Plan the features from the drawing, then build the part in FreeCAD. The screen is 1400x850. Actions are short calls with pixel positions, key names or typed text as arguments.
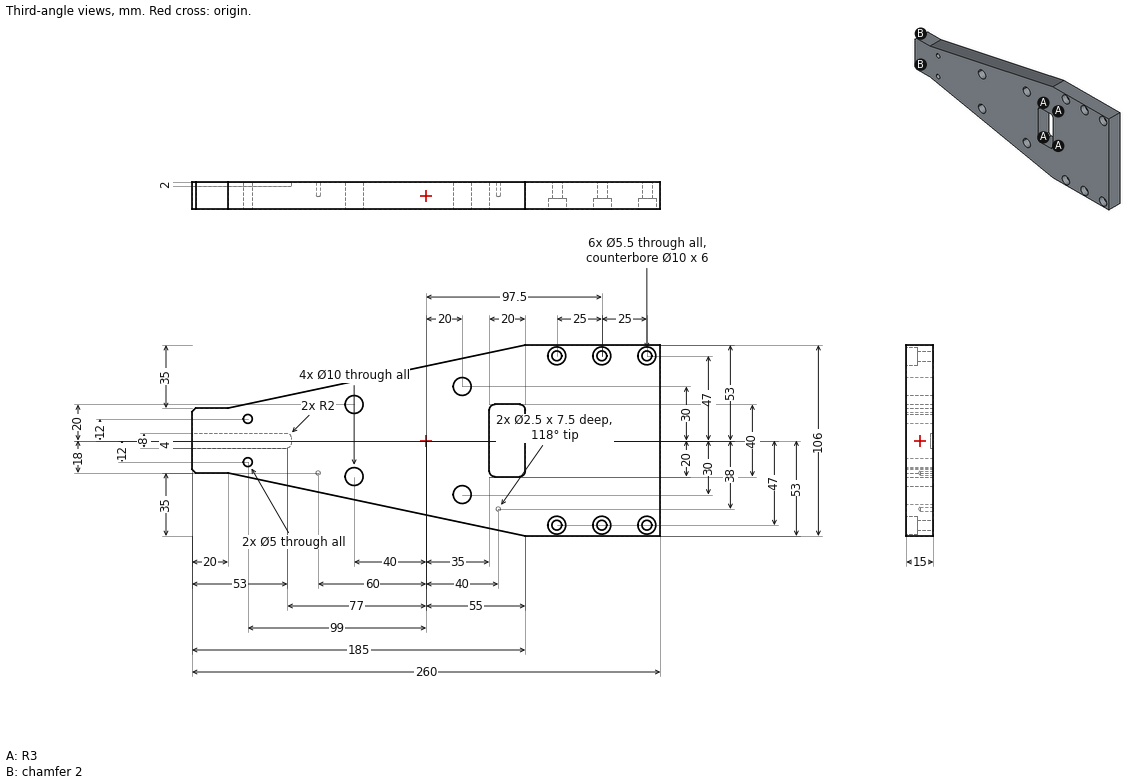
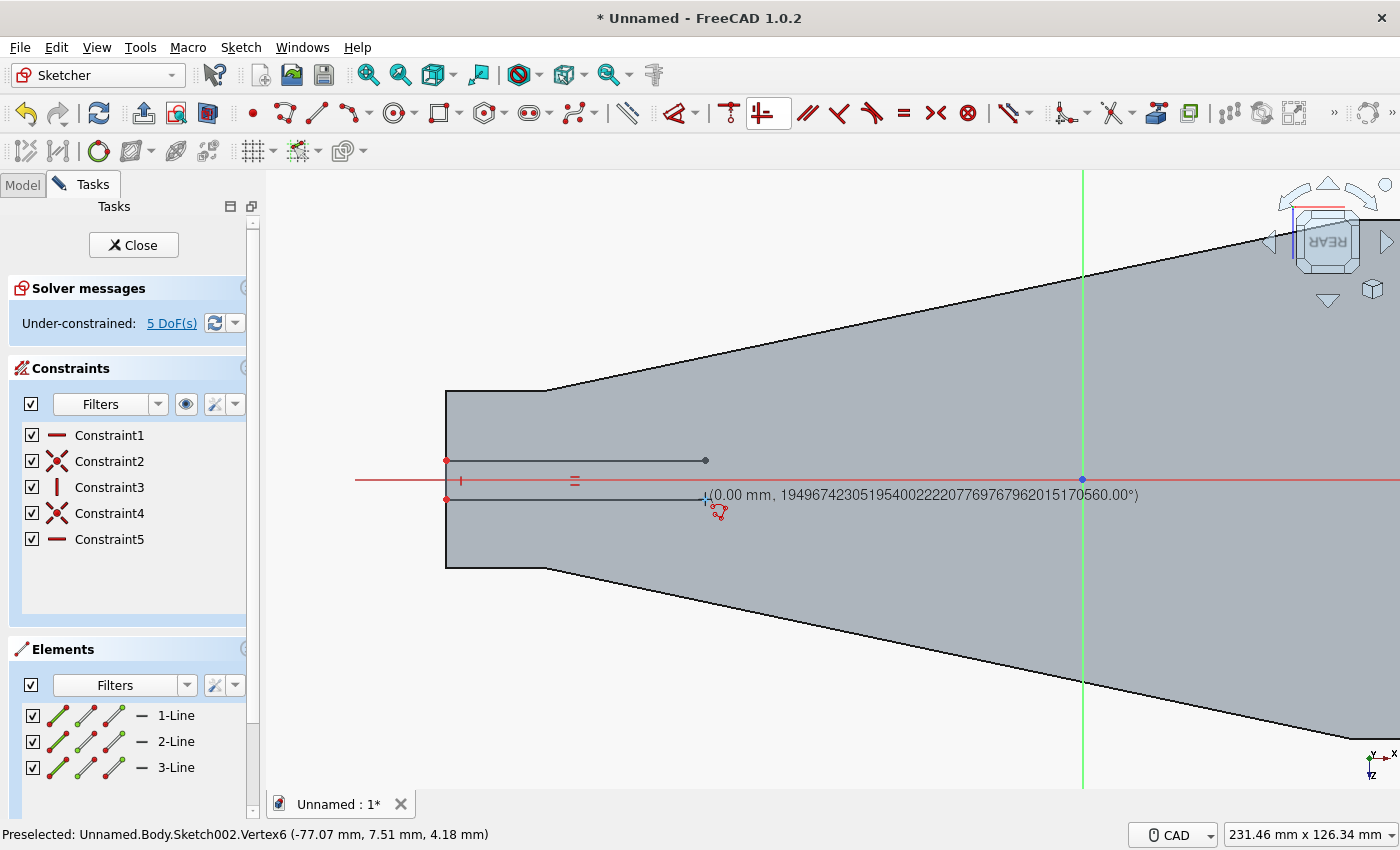
click(318, 114)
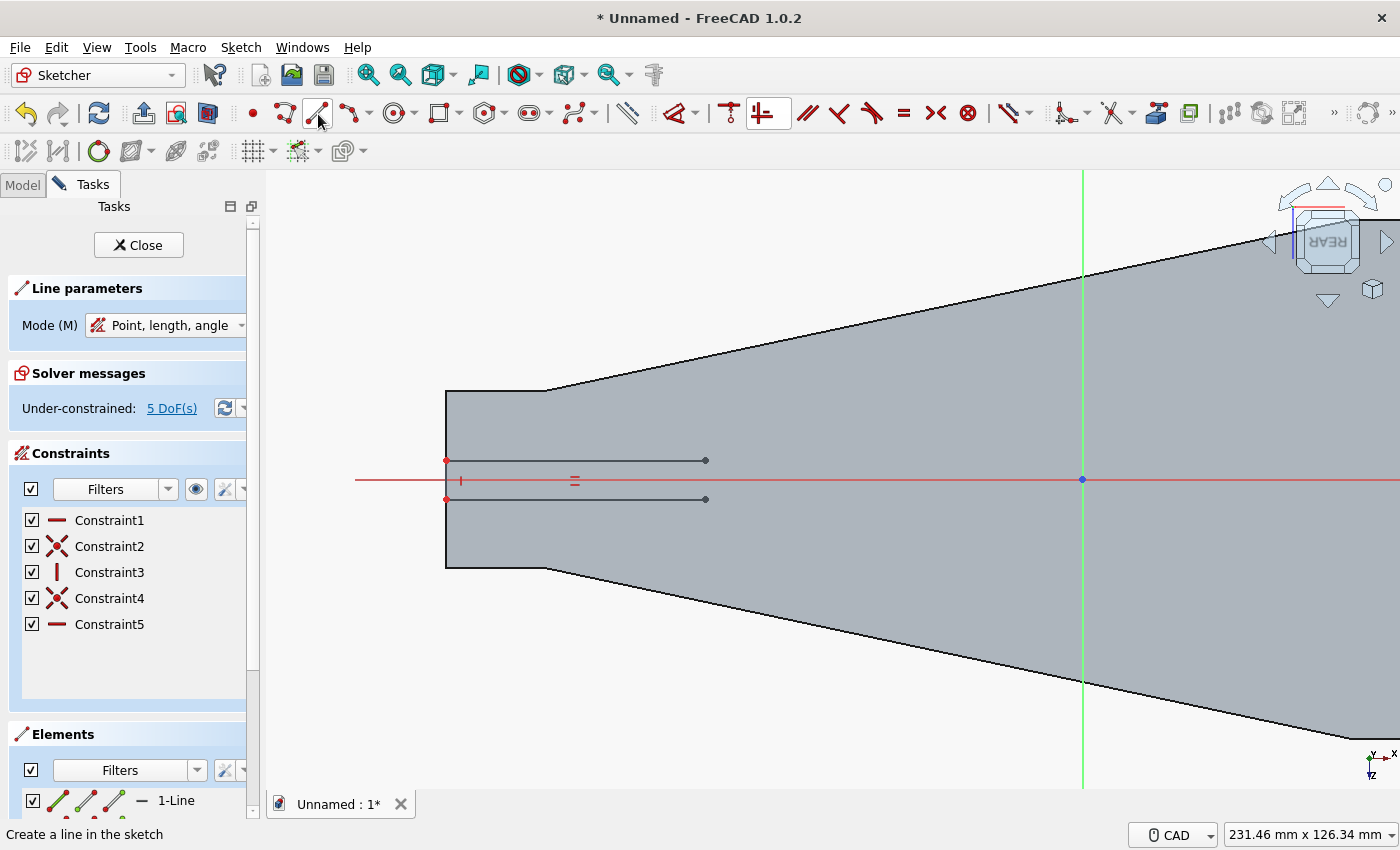
scroll(715, 489, up, 3)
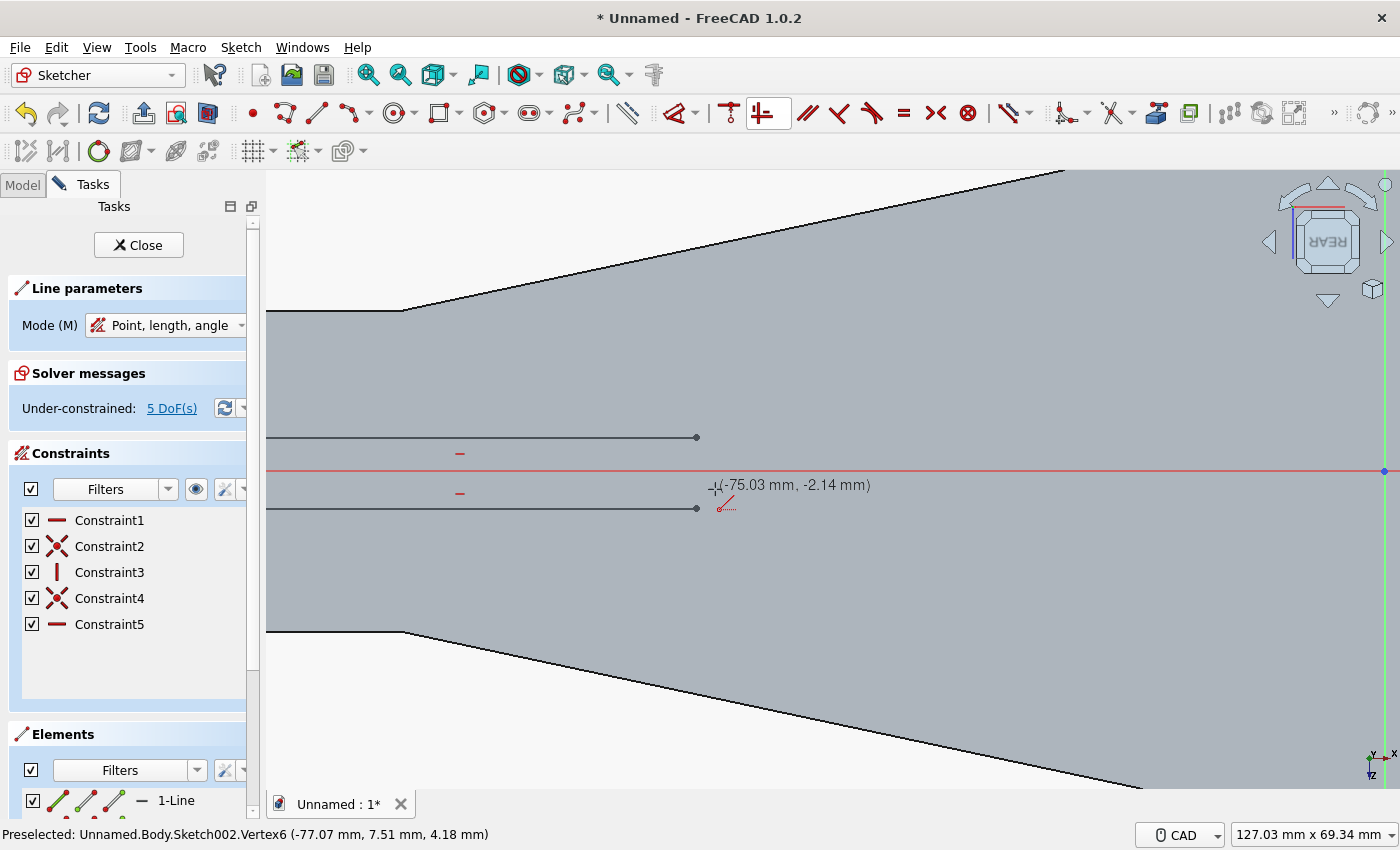
click(715, 489)
click(715, 453)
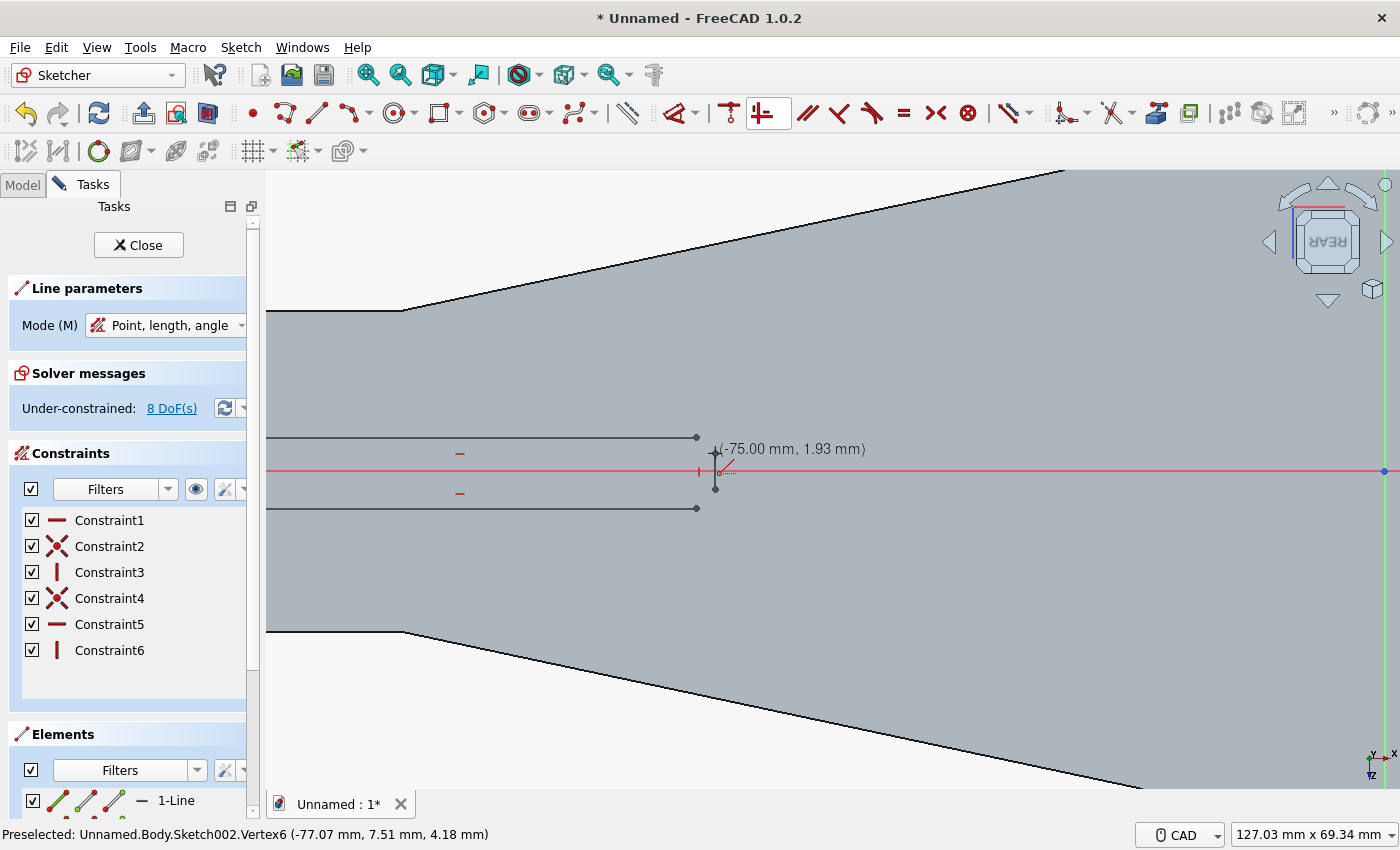
click(350, 114)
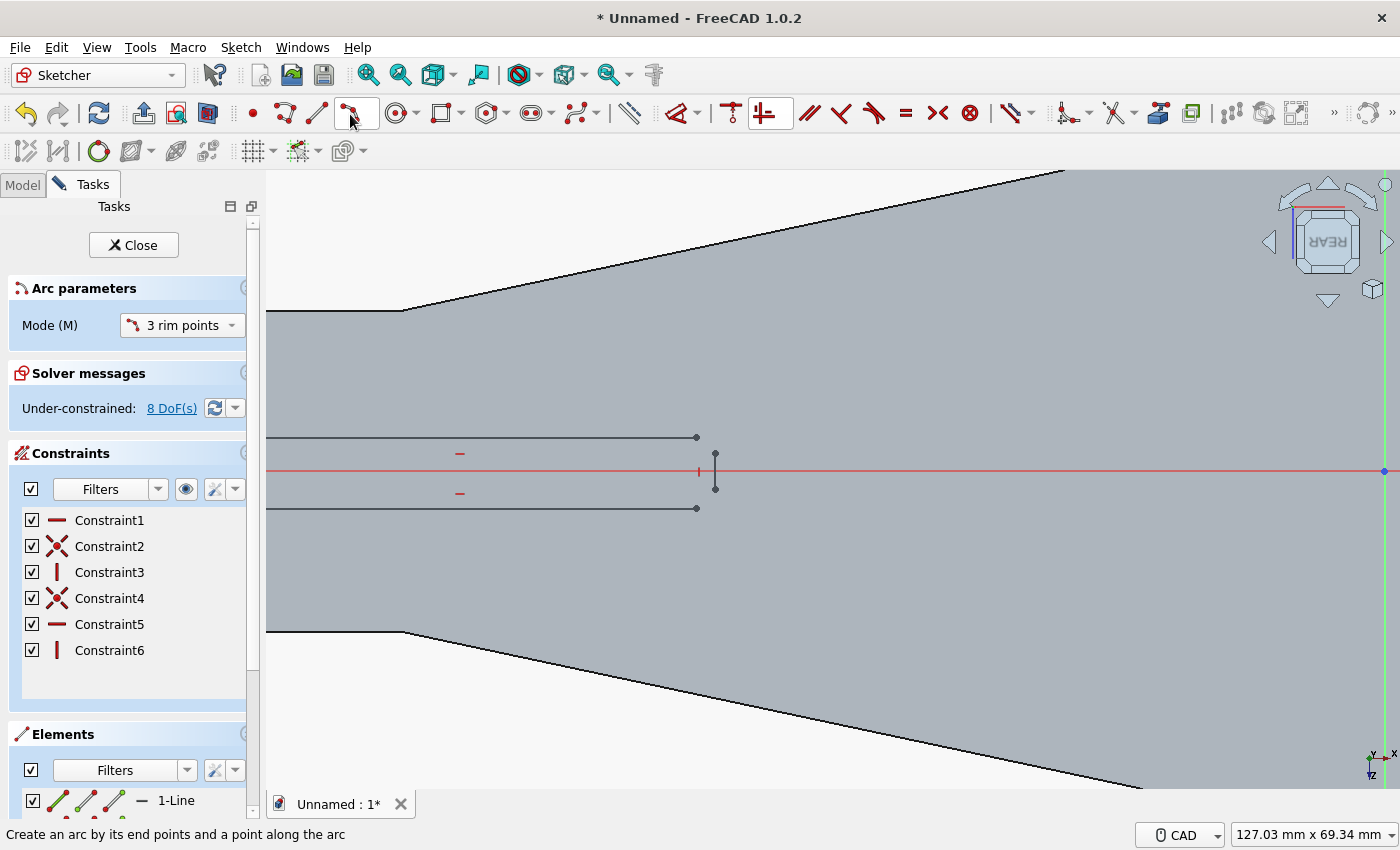
click(696, 509)
click(715, 490)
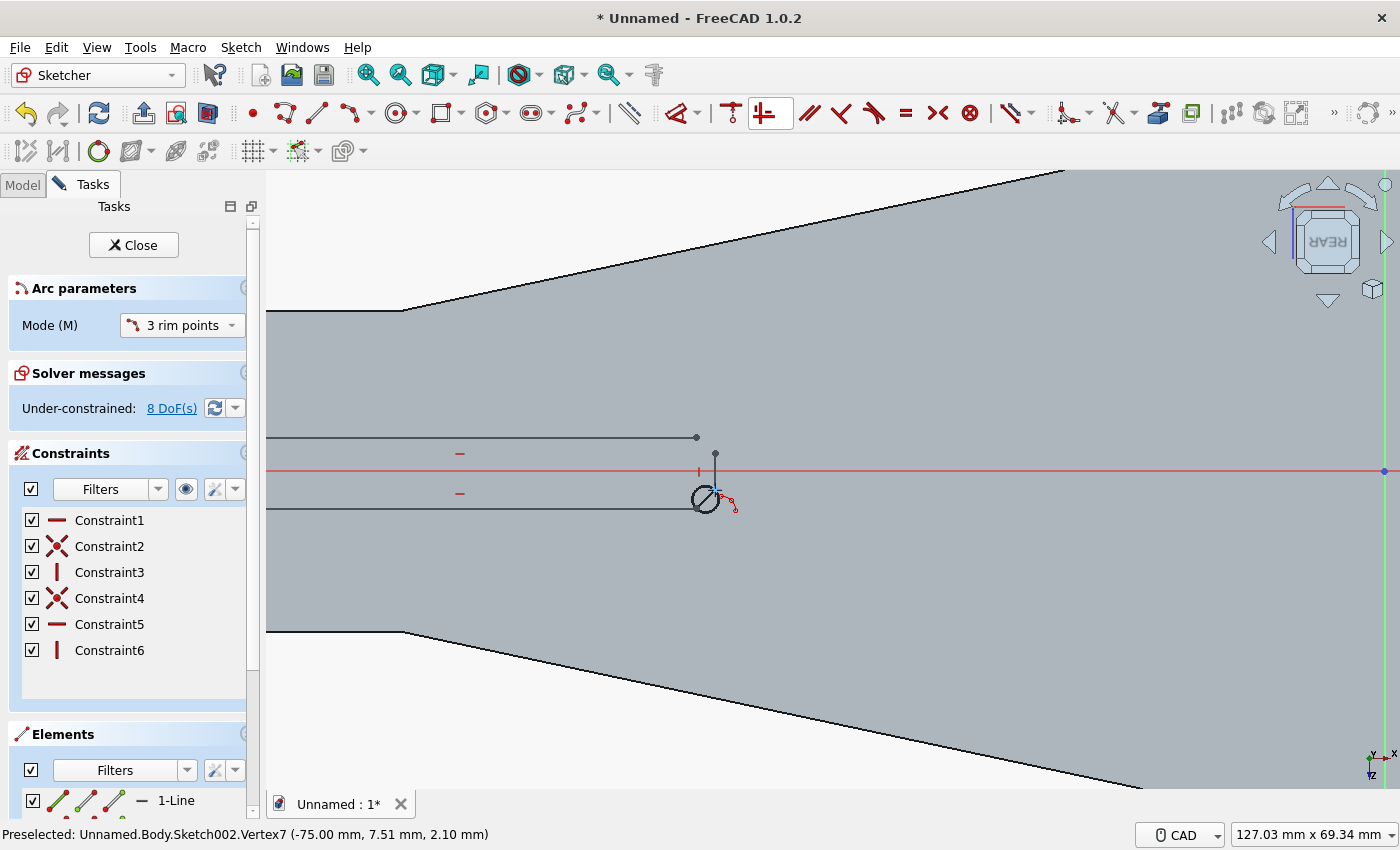
scroll(710, 502, up, 6)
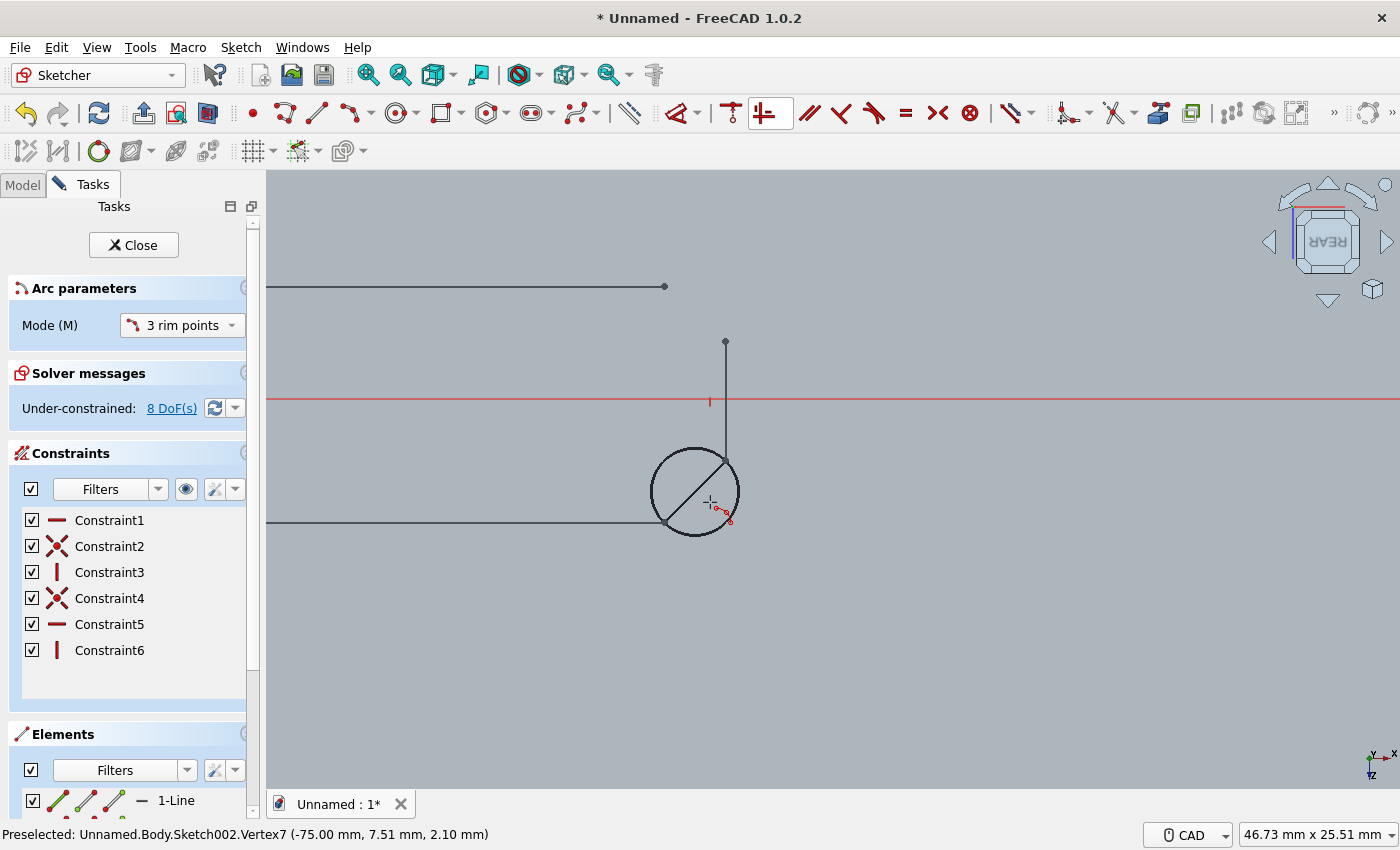
click(708, 500)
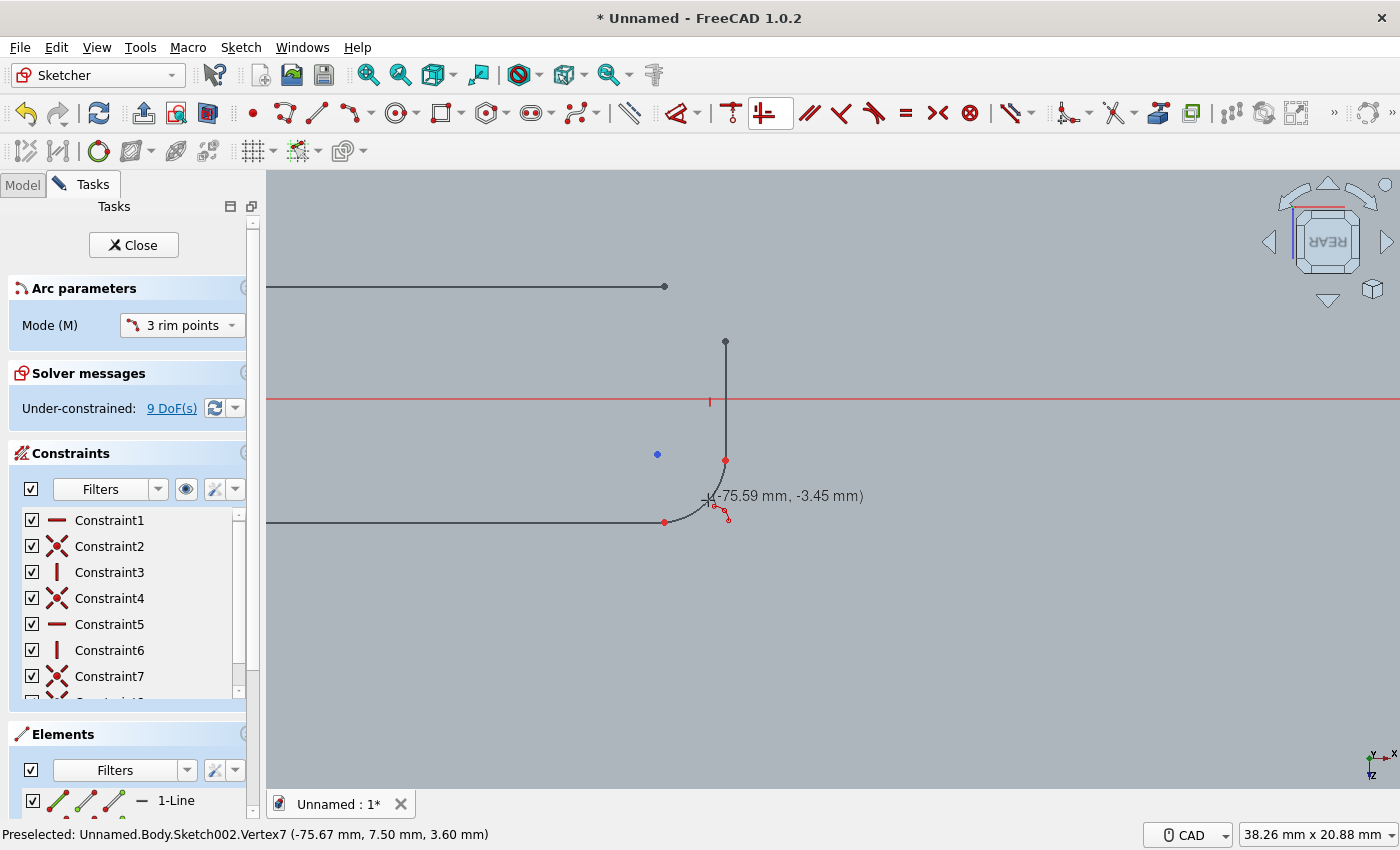
scroll(714, 495, down, 9)